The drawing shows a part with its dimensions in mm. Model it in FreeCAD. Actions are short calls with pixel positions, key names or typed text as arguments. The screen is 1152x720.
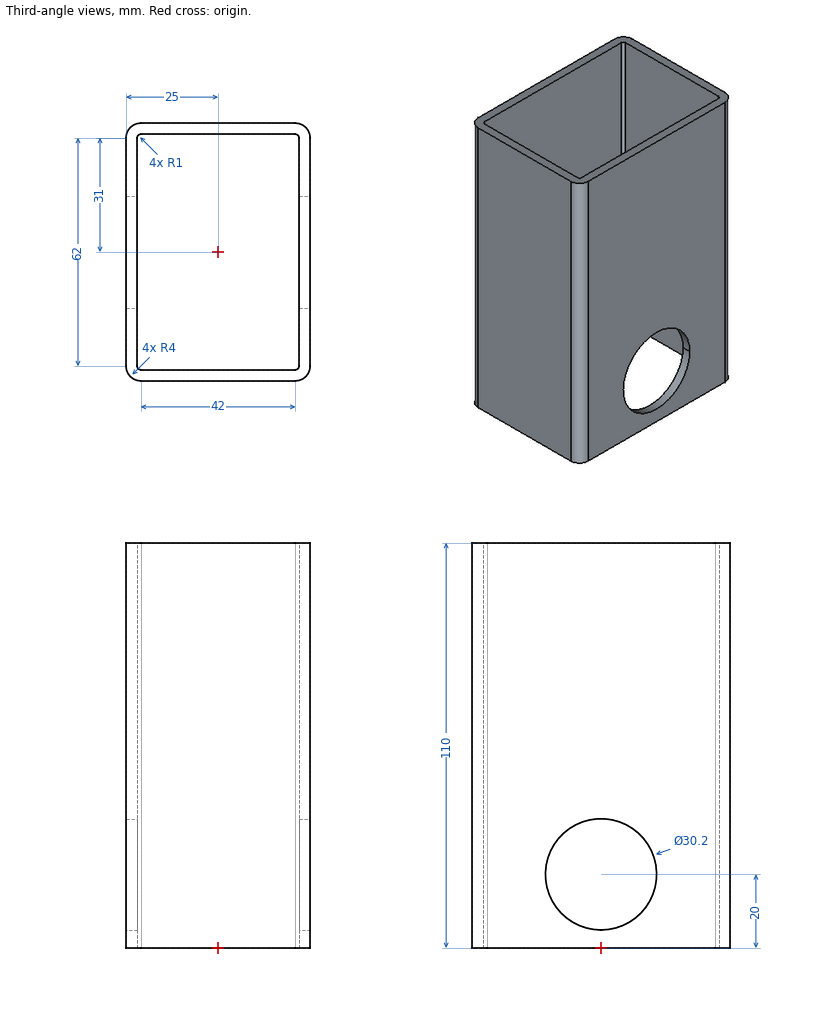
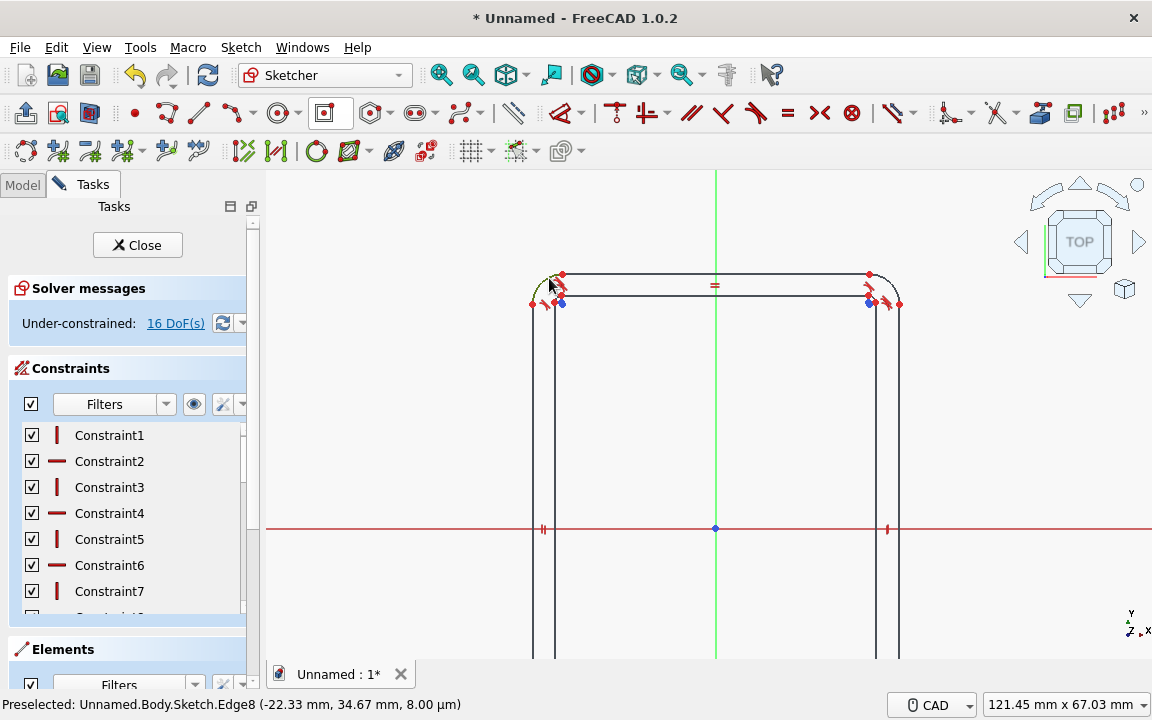
scroll(557, 298, up, 5)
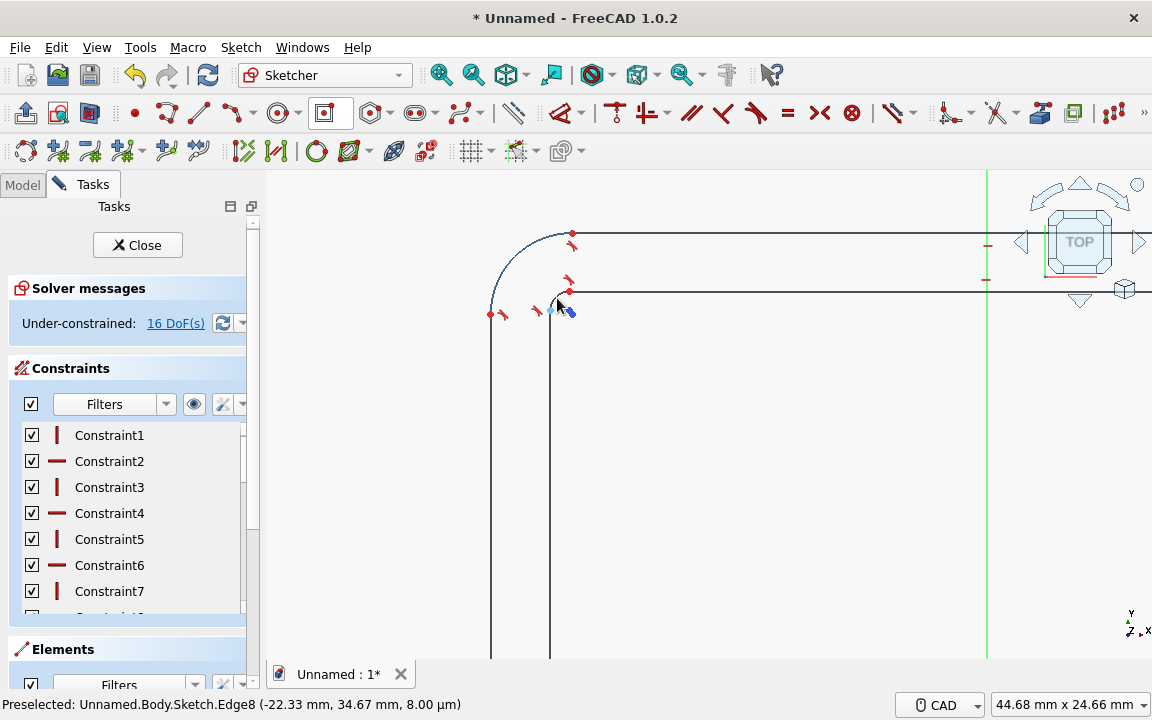
click(556, 297)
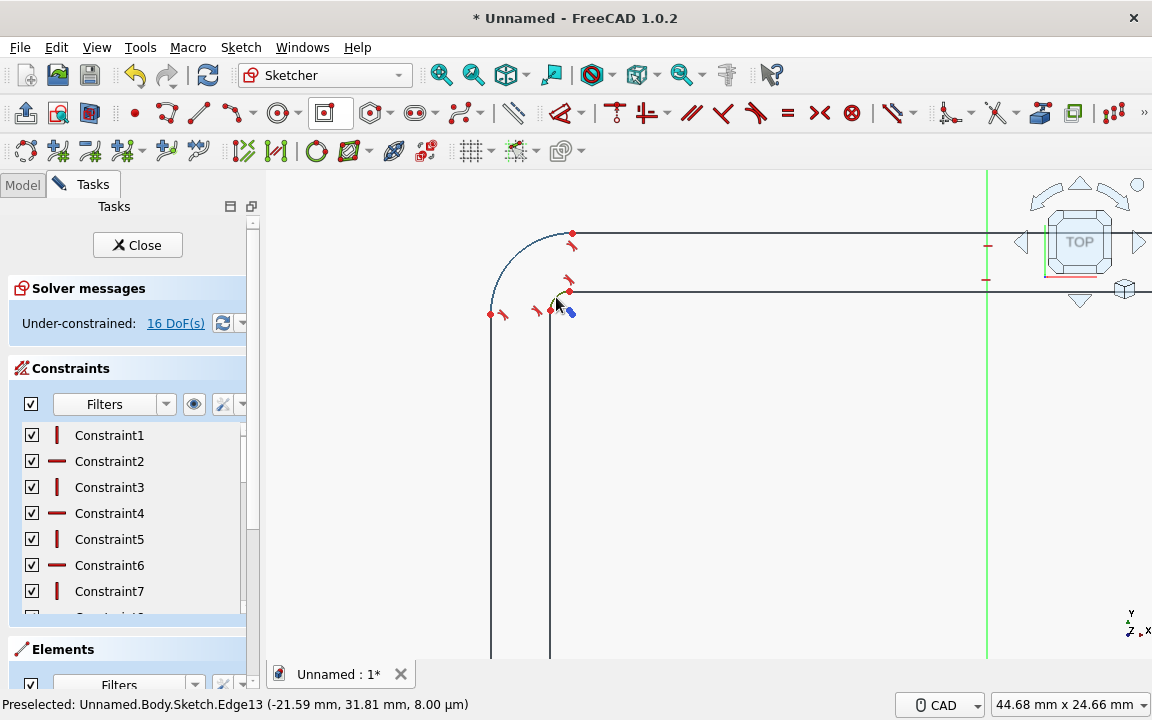
key(c)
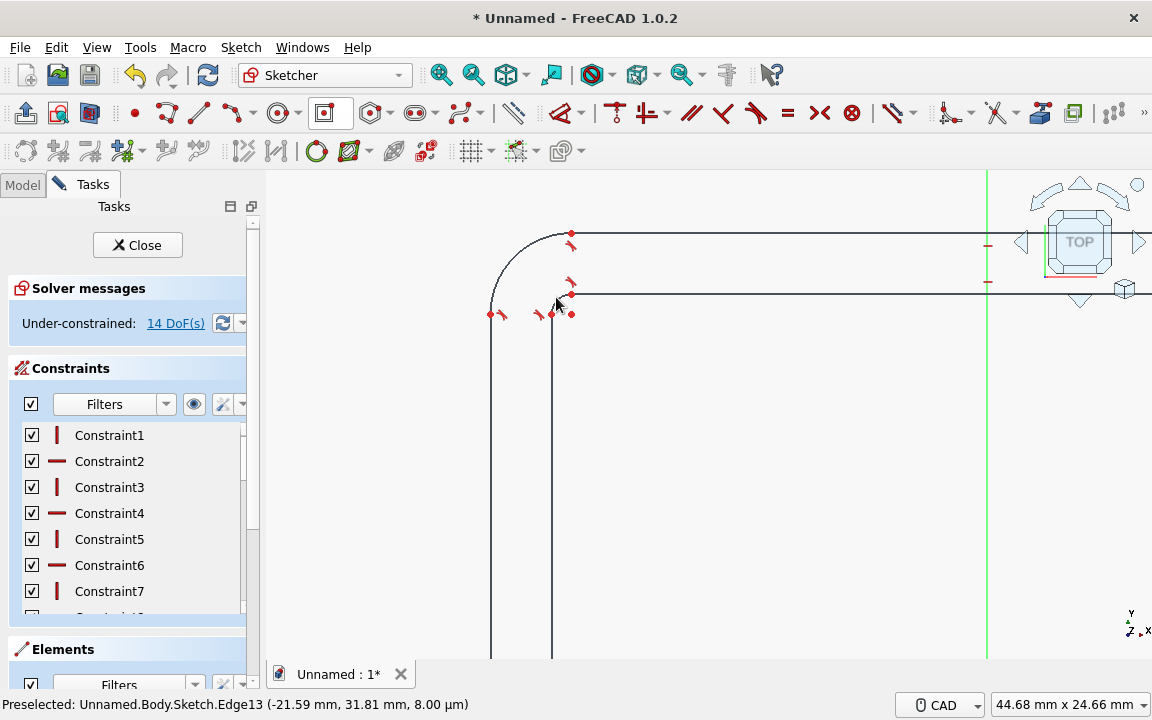
scroll(553, 285, down, 8)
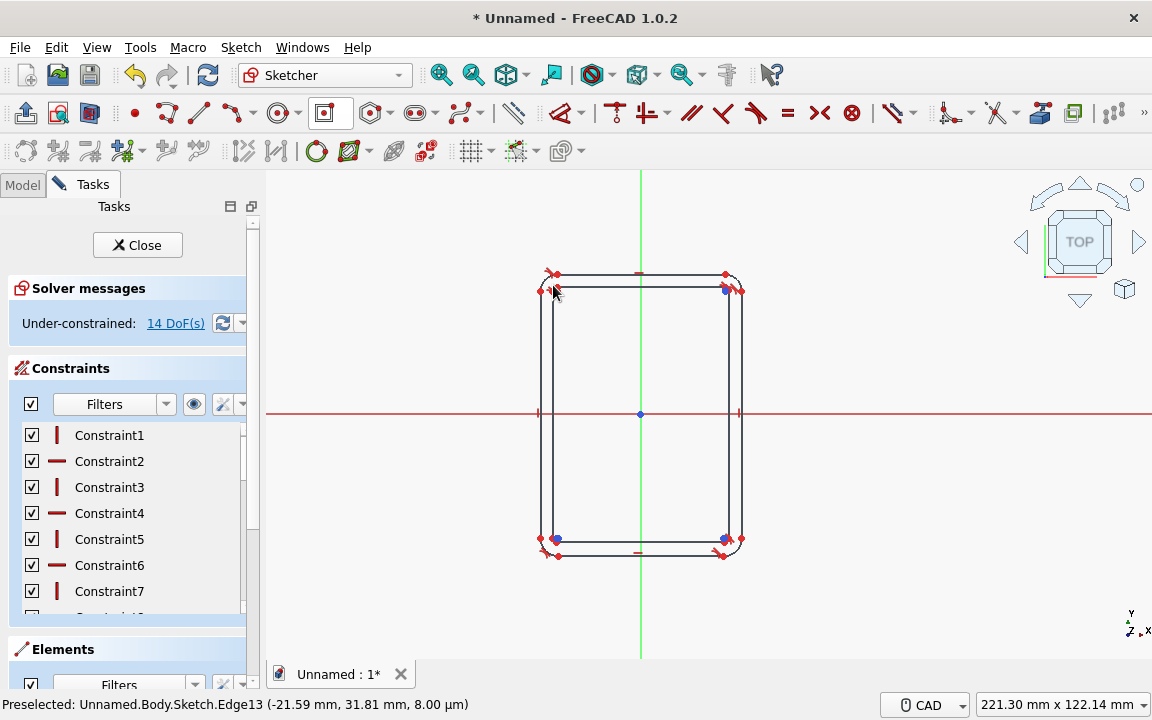
scroll(740, 284, up, 3)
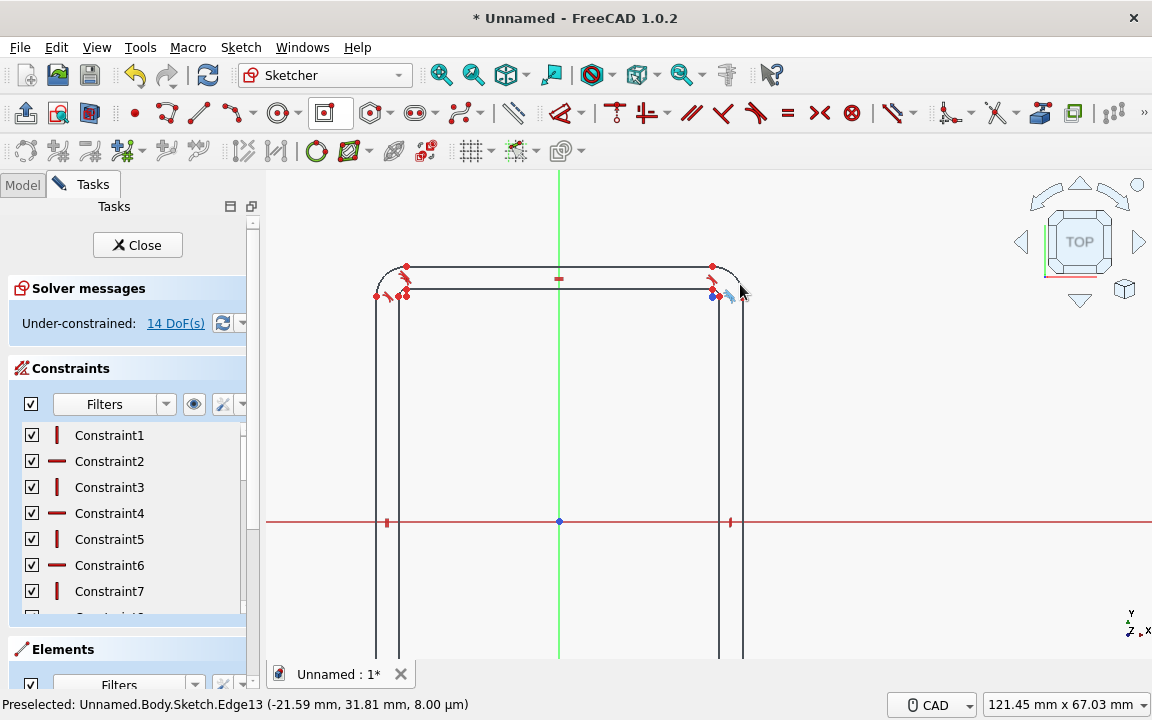
click(740, 283)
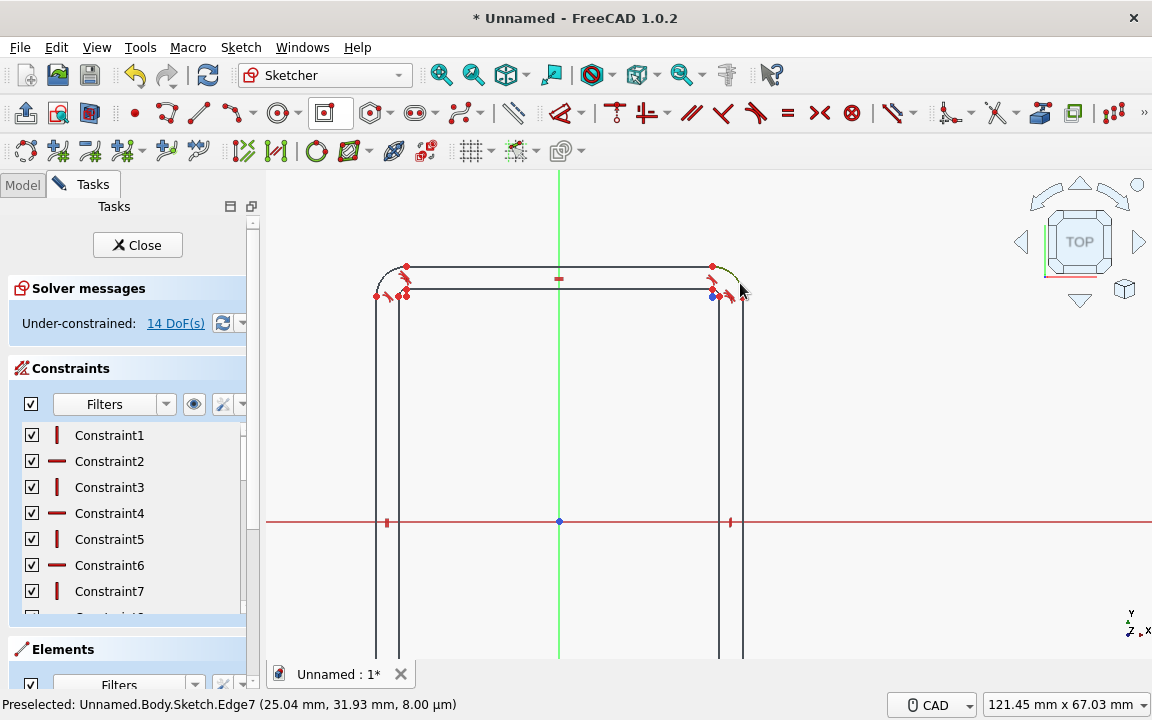
scroll(717, 291, up, 5)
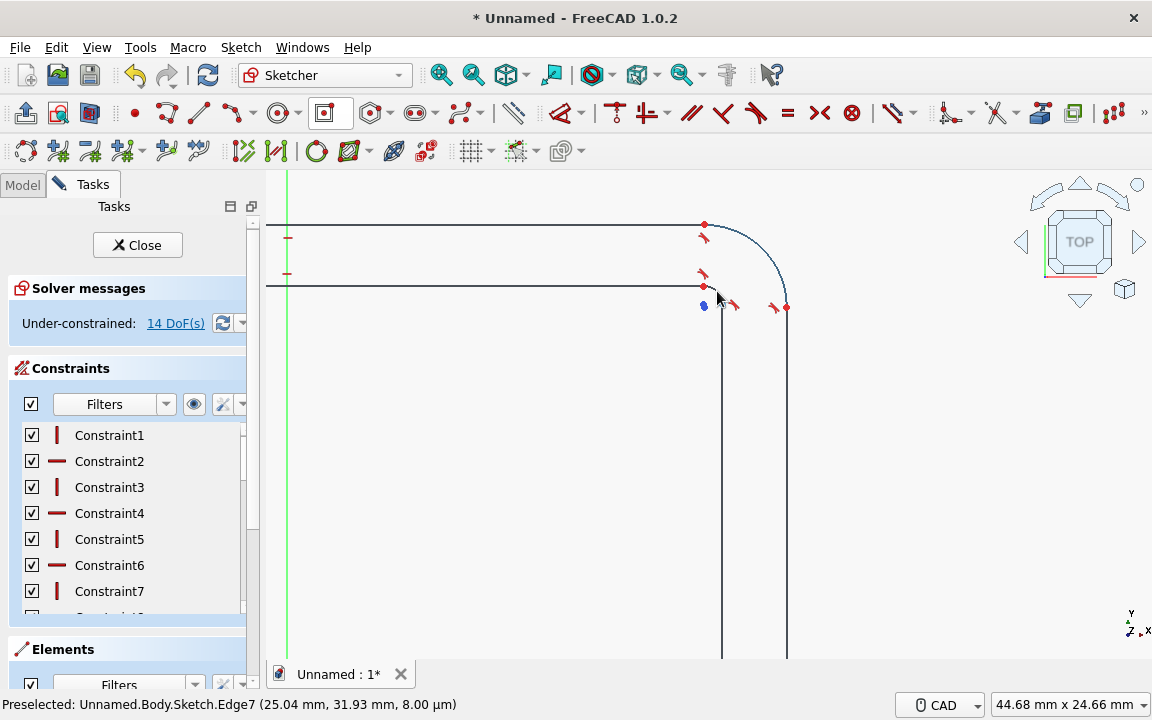
click(717, 291)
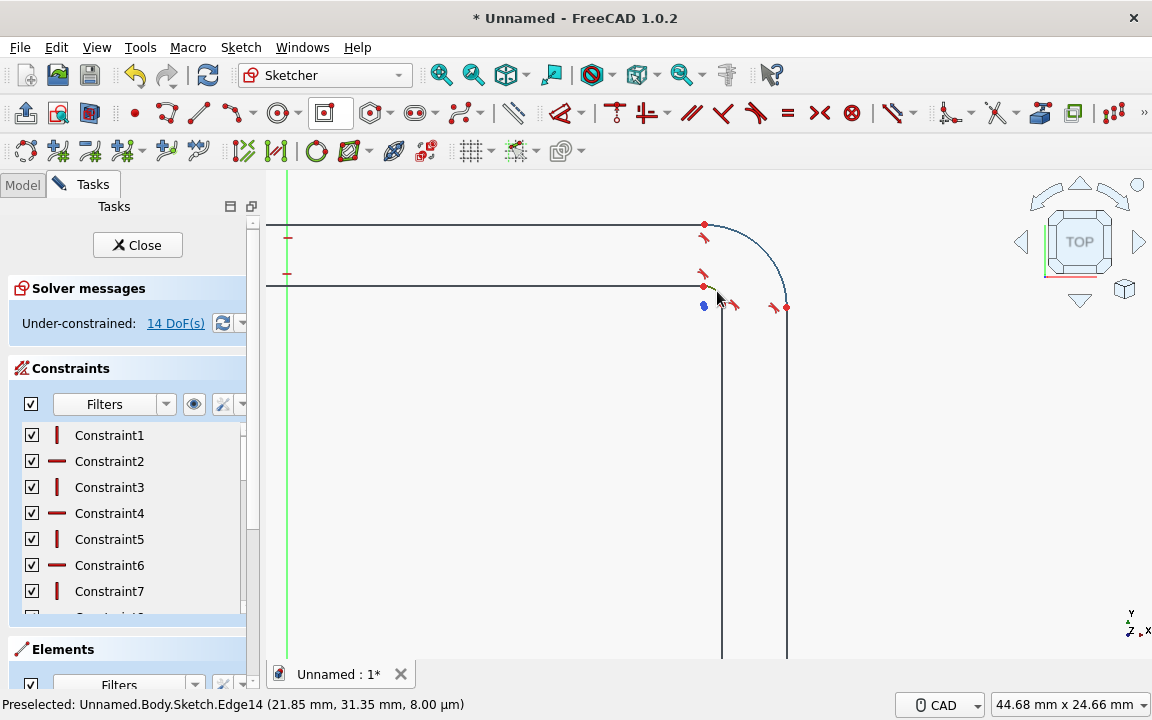
click(616, 114)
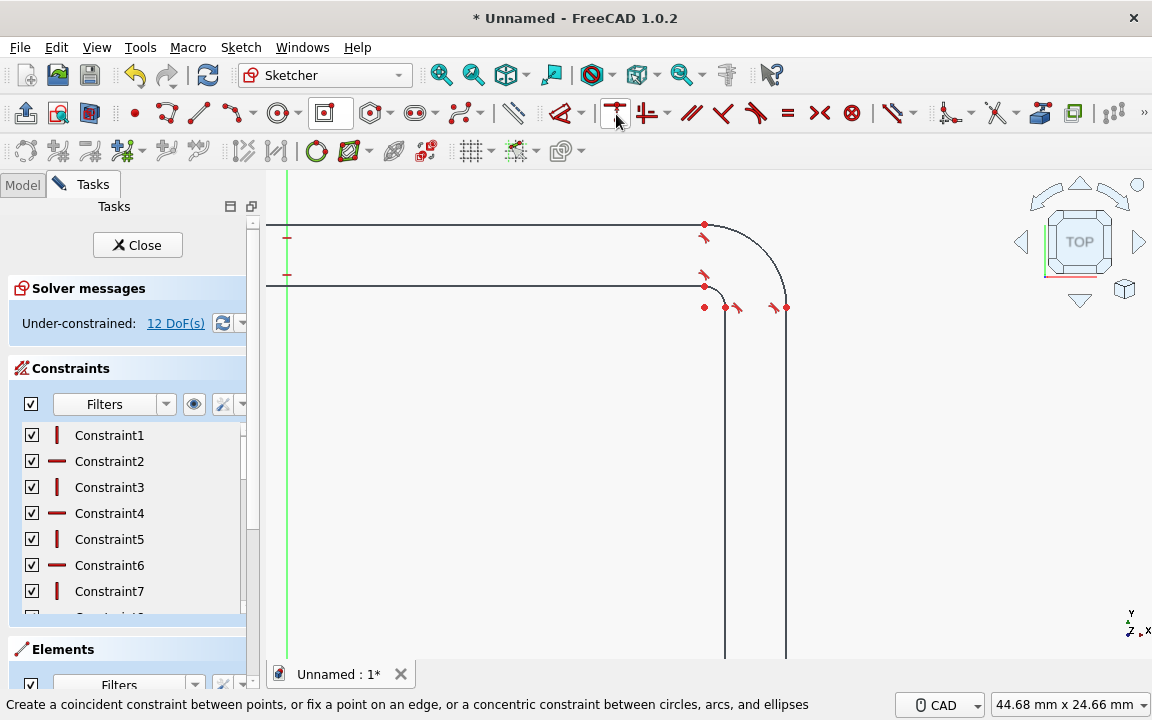
scroll(730, 287, down, 8)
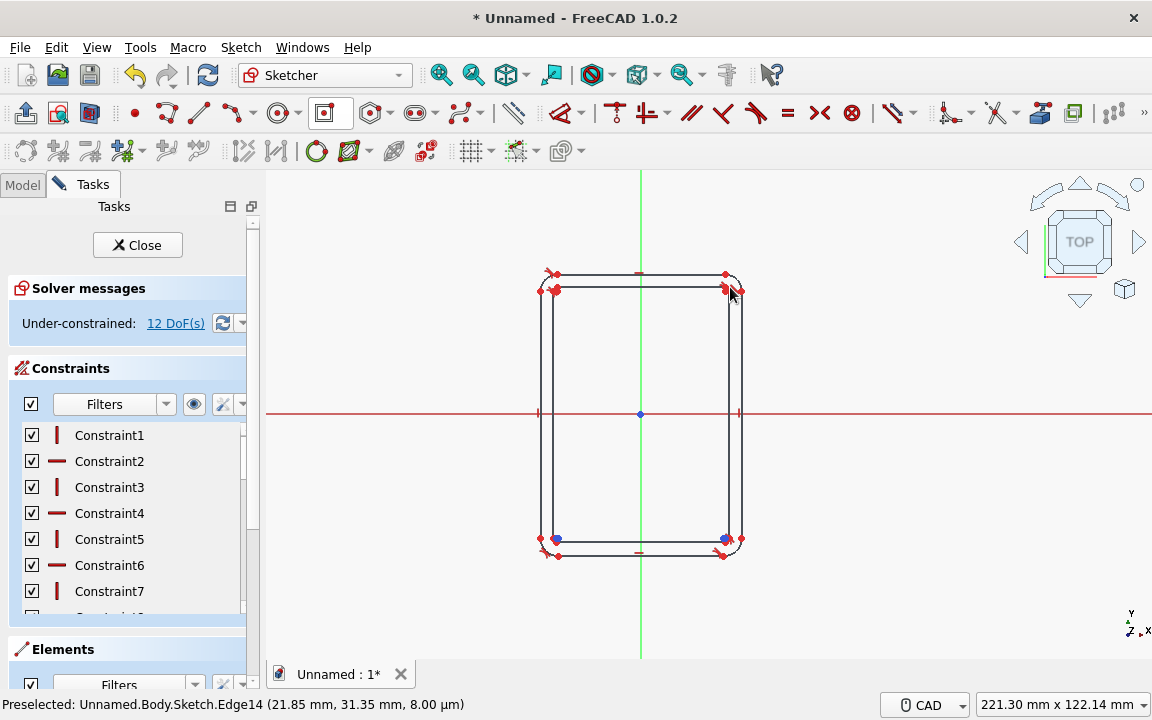
scroll(732, 554, up, 3)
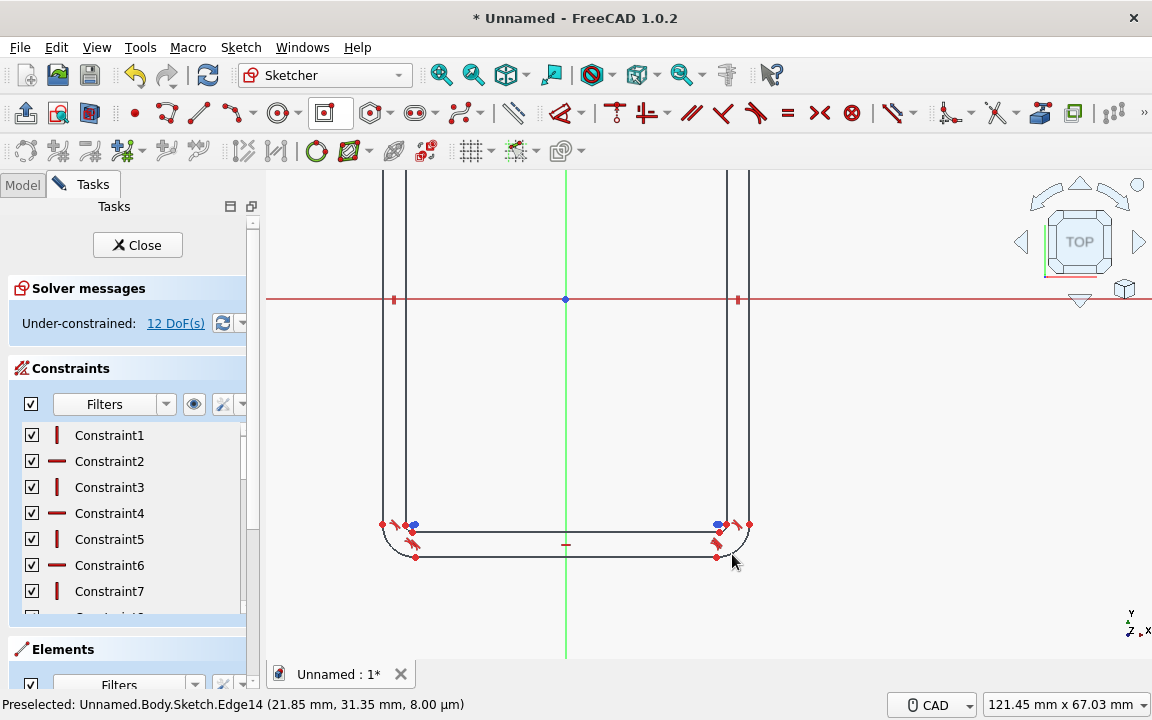
click(732, 554)